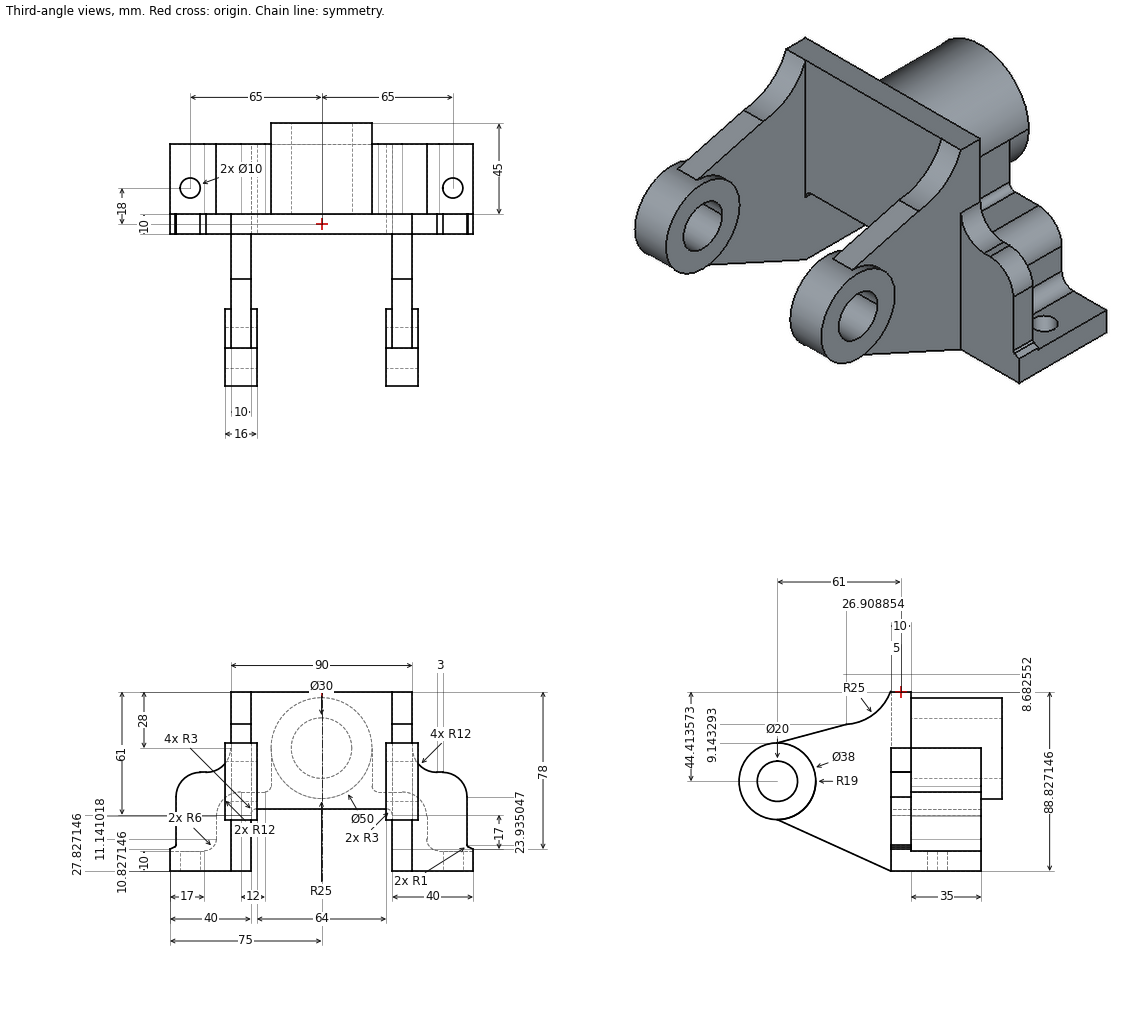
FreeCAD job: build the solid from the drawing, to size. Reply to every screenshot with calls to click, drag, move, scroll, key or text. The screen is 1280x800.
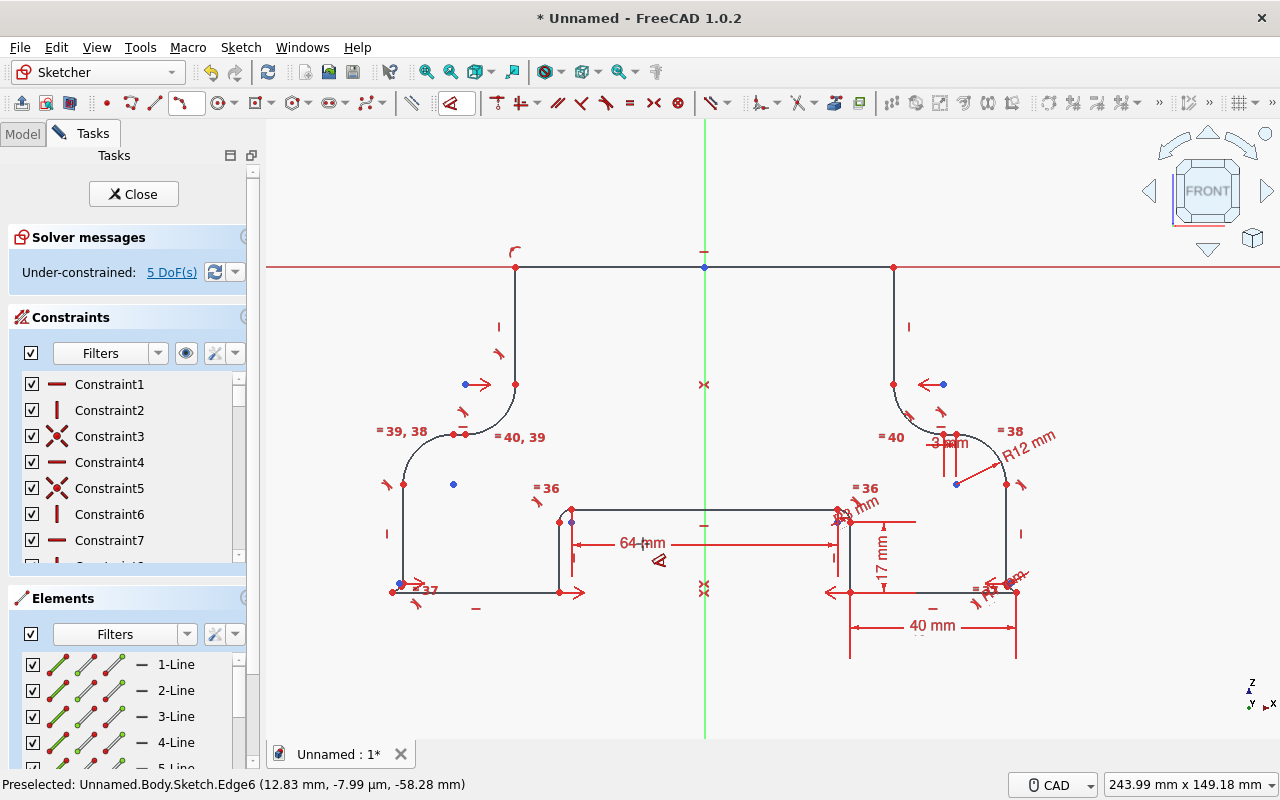
click(509, 593)
click(476, 627)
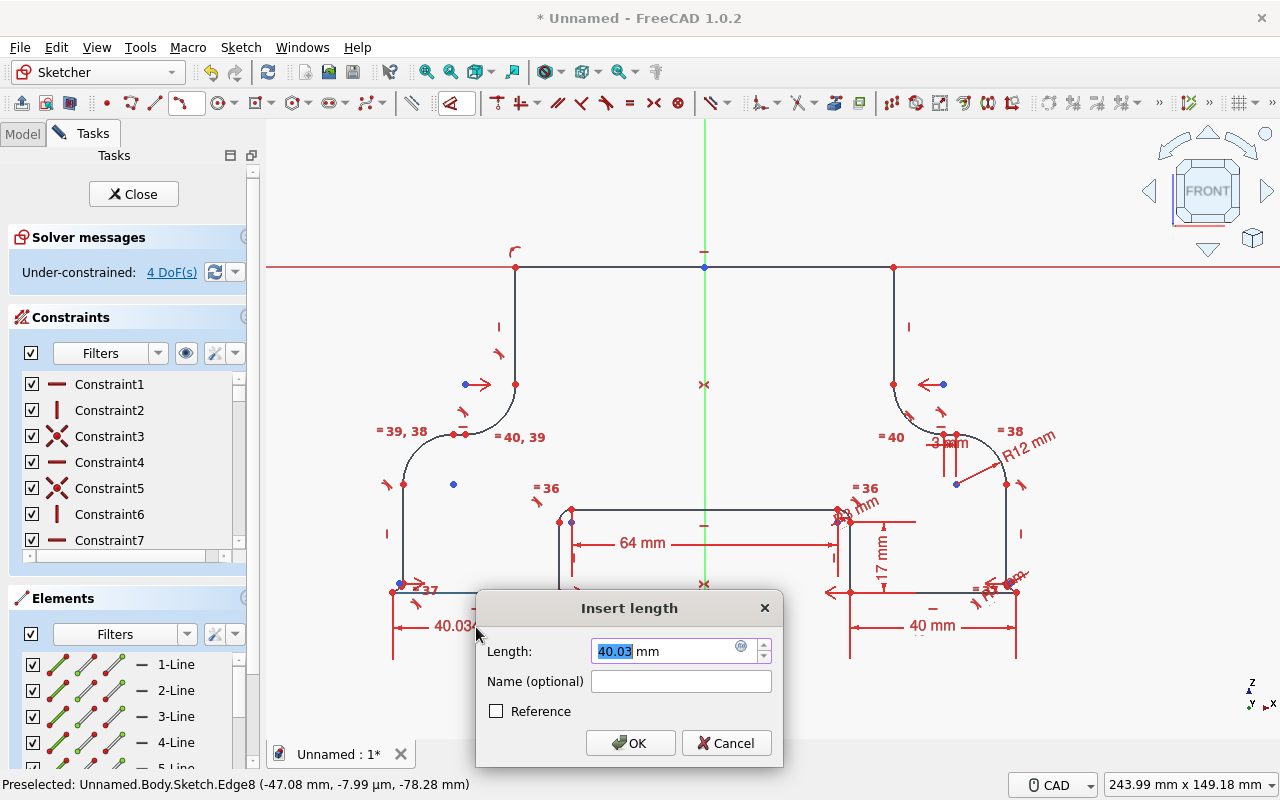
text(40)
key(Return)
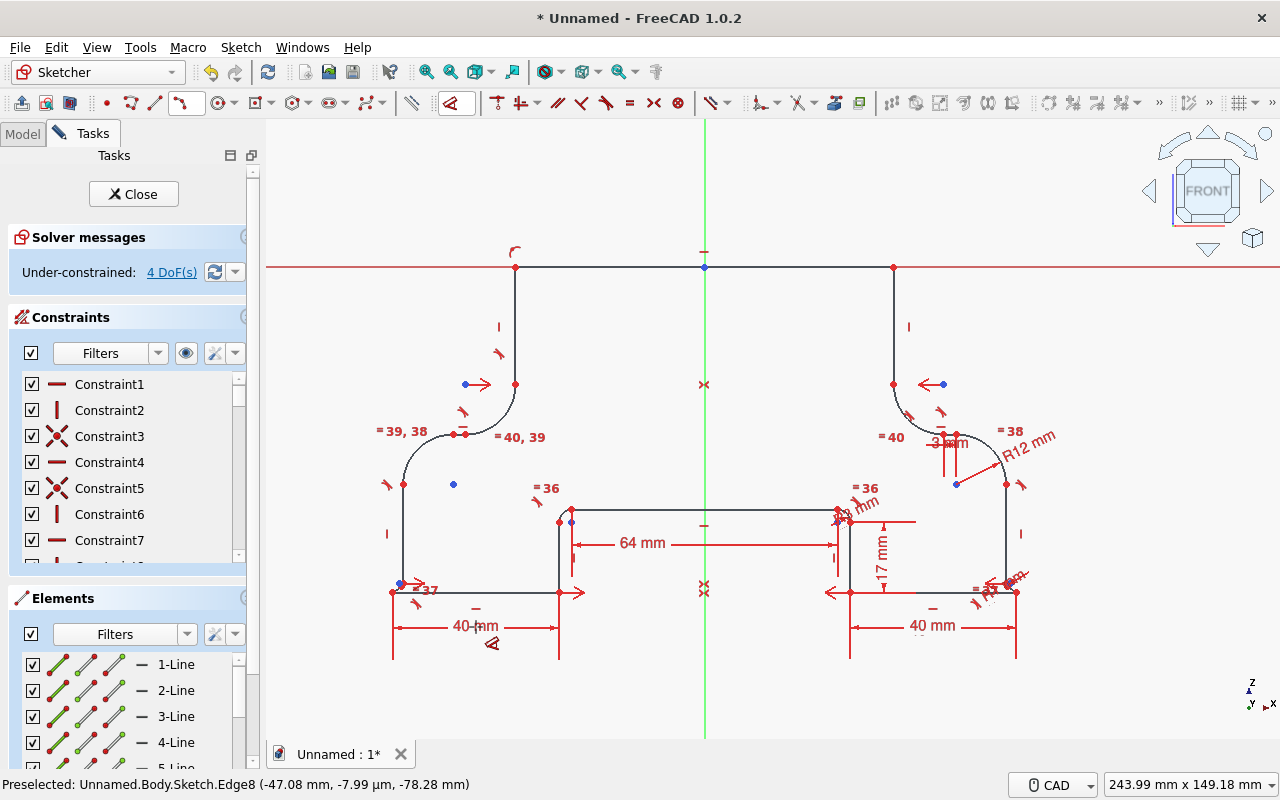
click(515, 349)
click(481, 326)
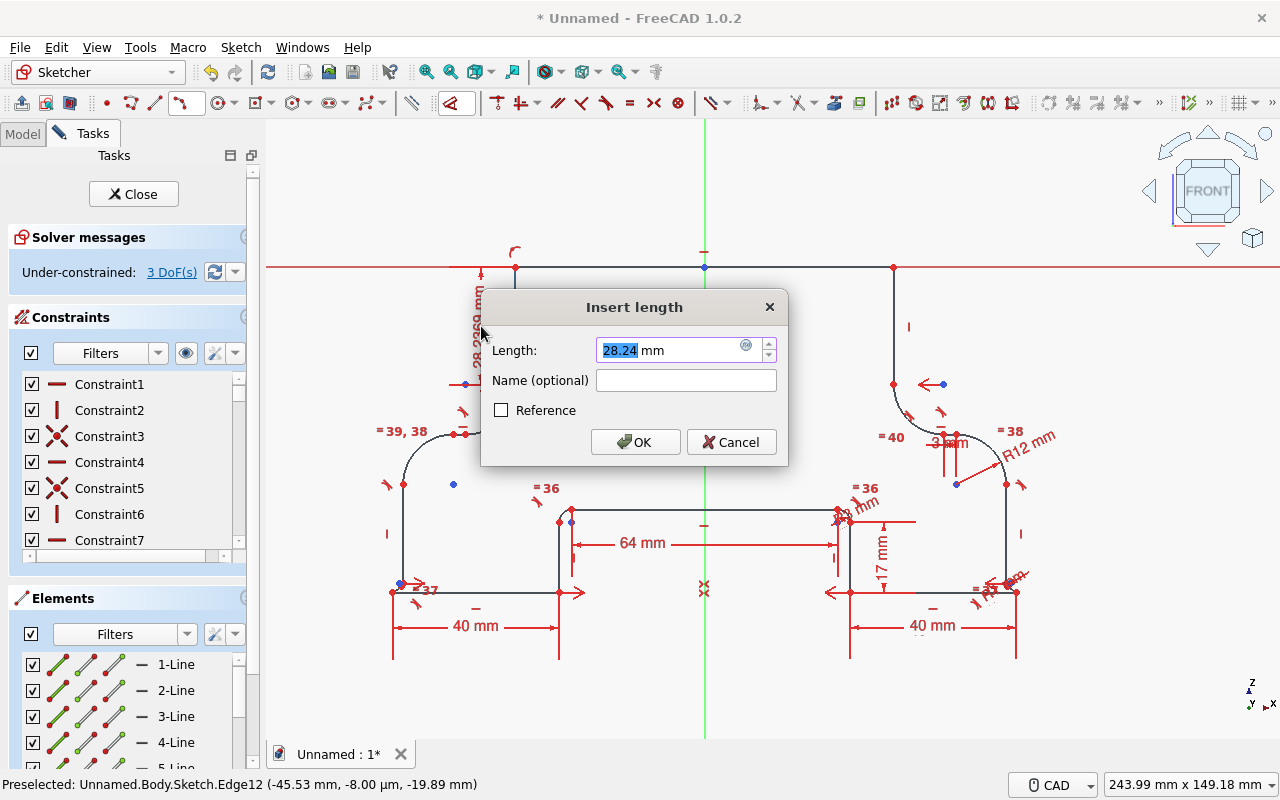
text(28)
key(Return)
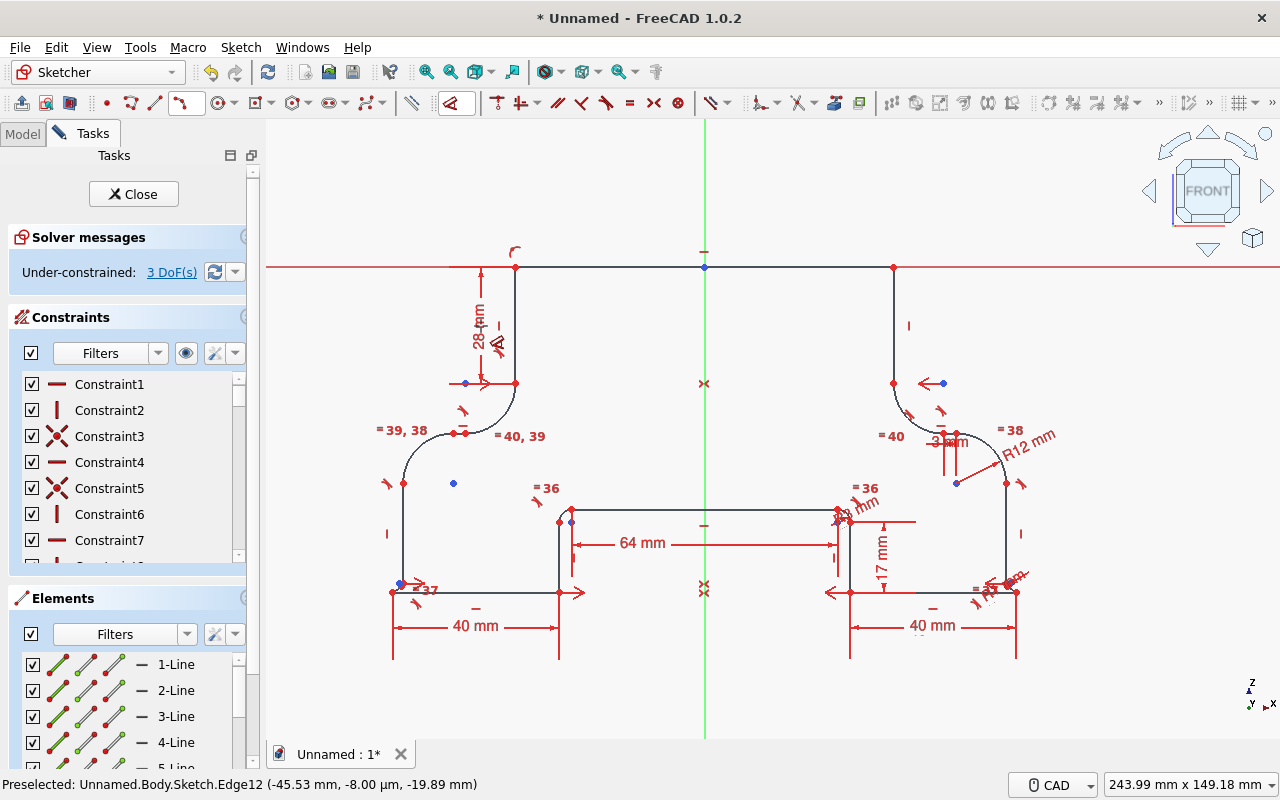
click(629, 267)
click(618, 233)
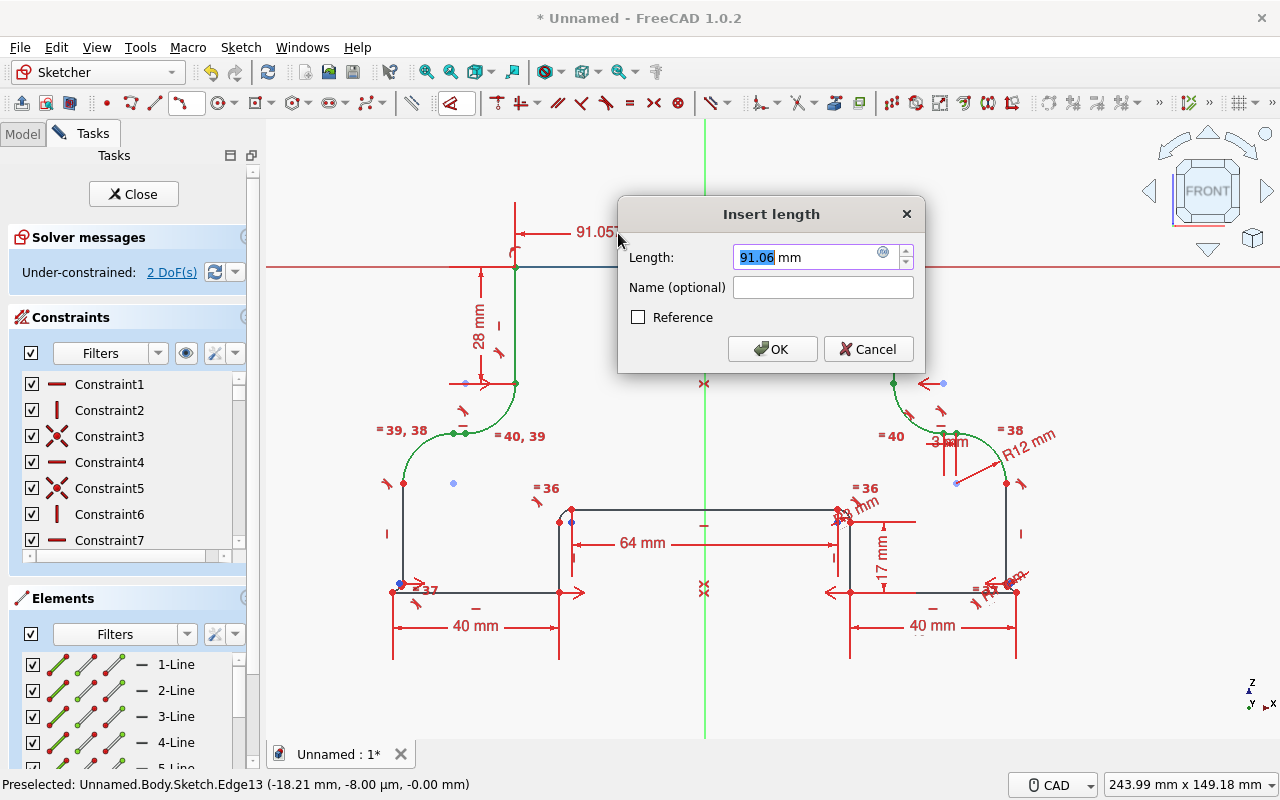
text(90)
key(Return)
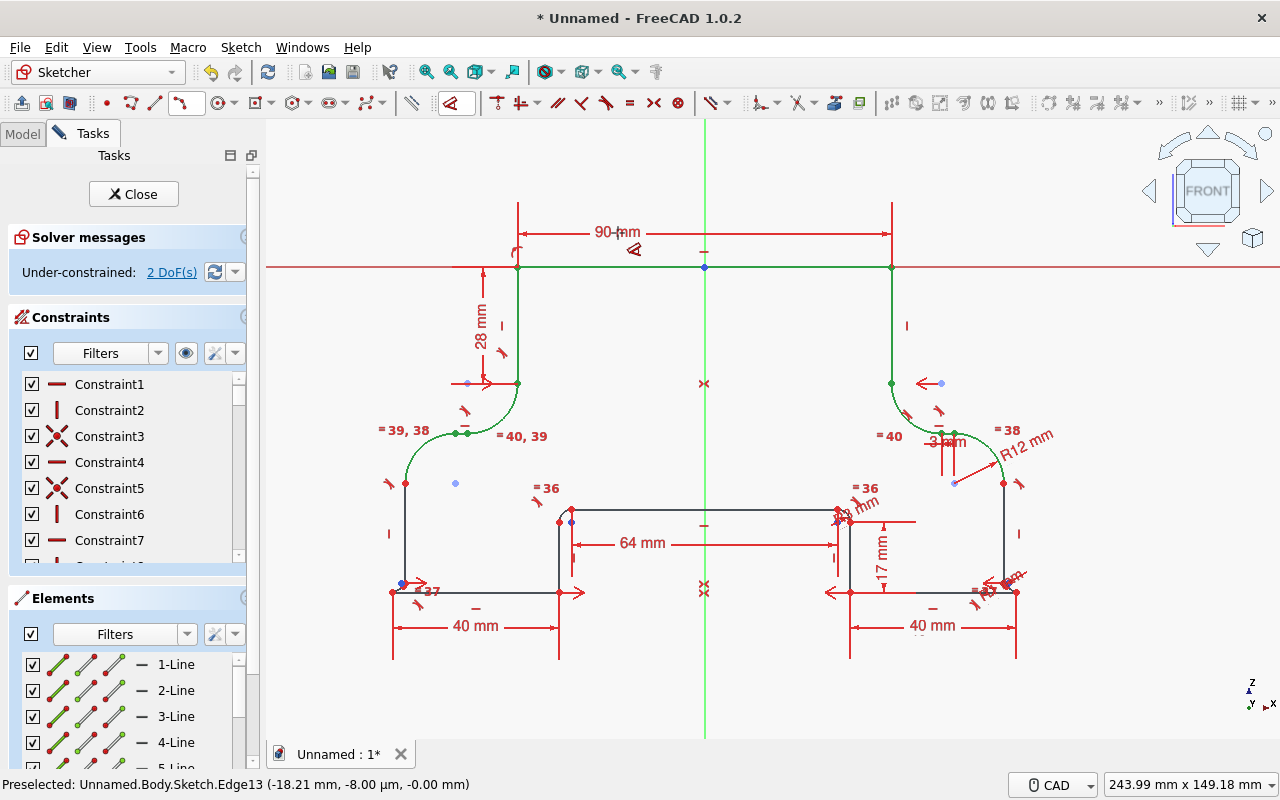
click(1016, 593)
click(1050, 355)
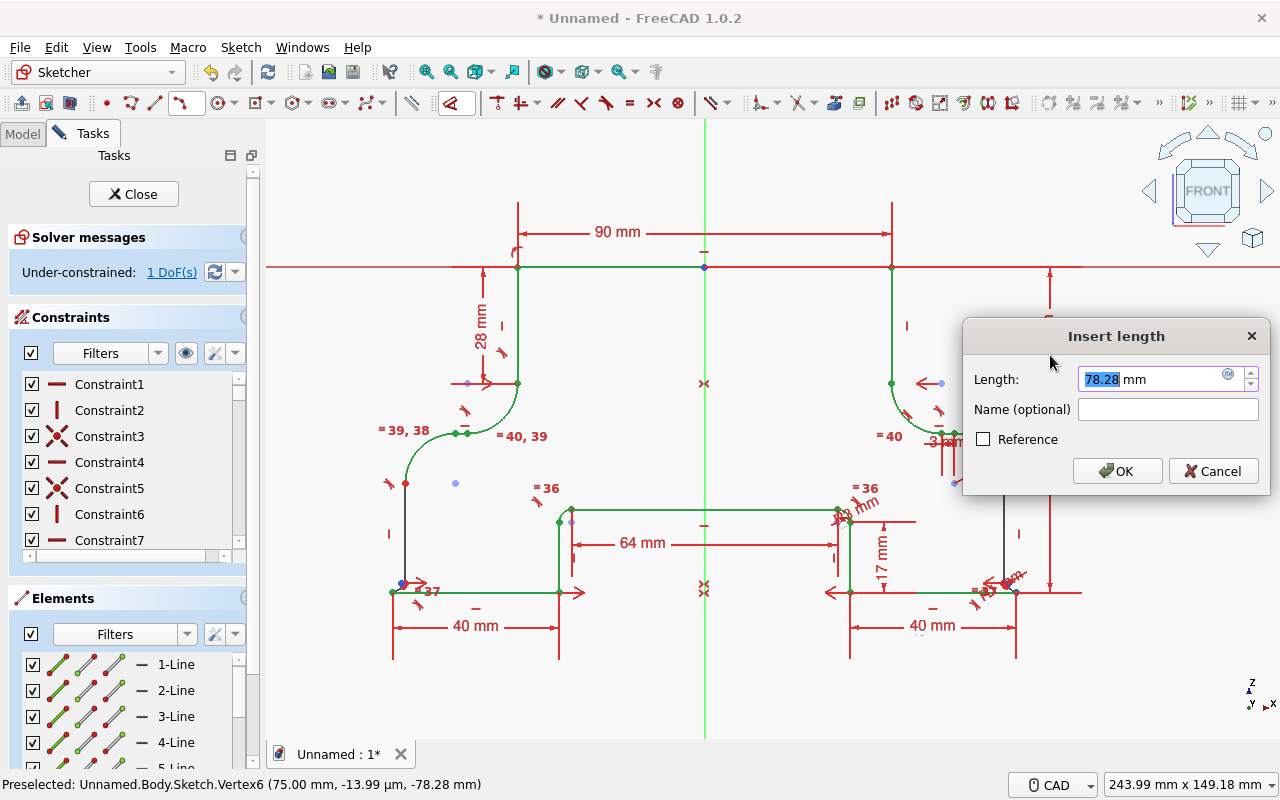
text(78)
key(Return)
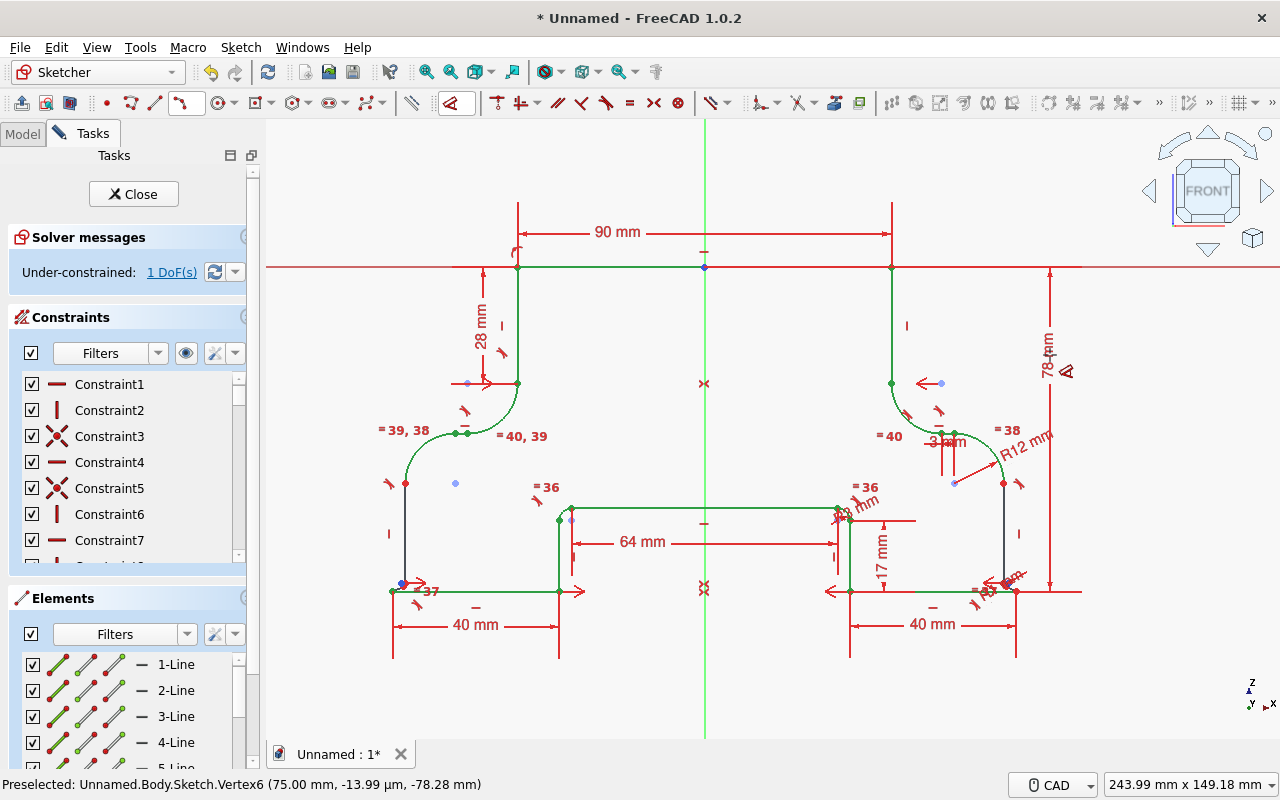
click(1004, 513)
click(1038, 533)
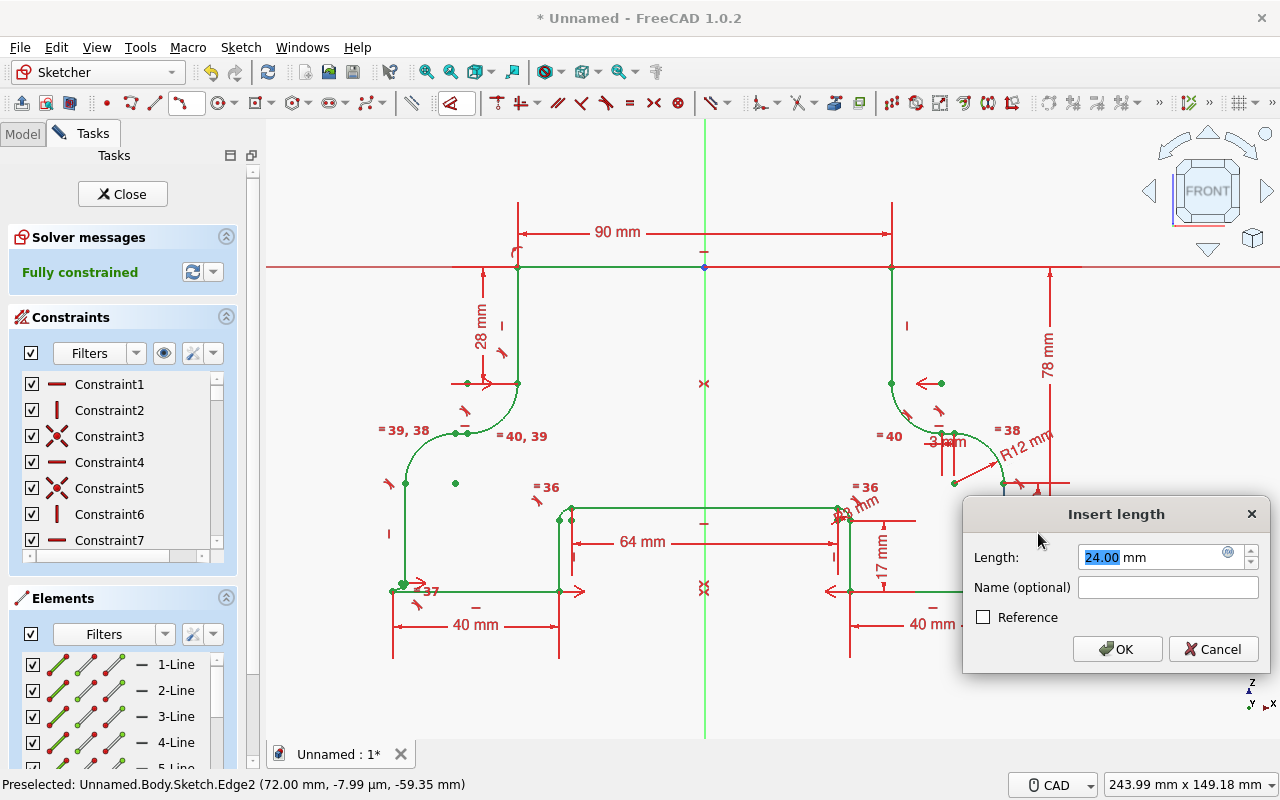
text(23.935047)
key(Return)
key(Escape)